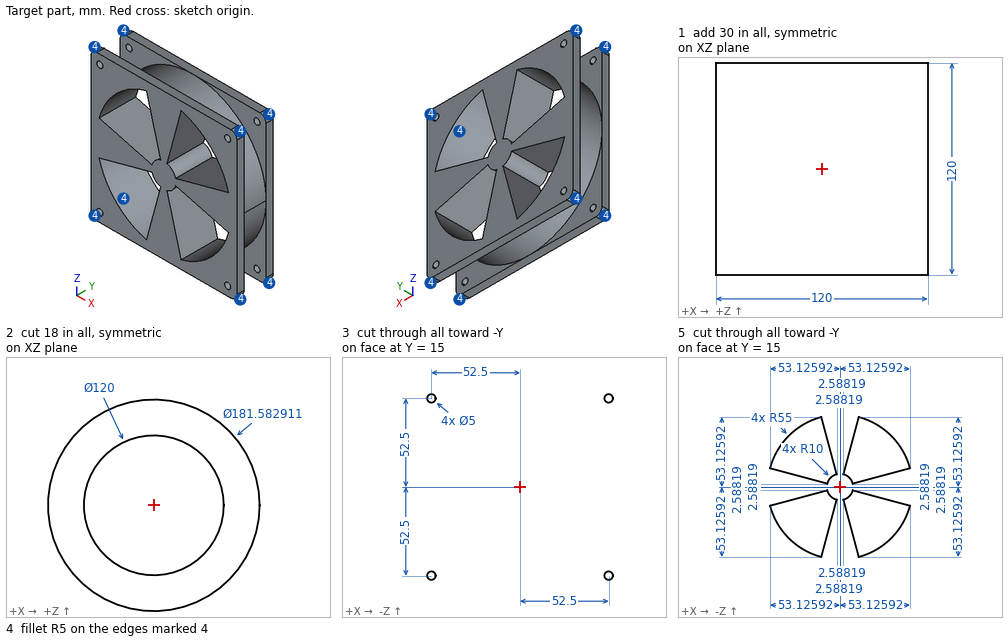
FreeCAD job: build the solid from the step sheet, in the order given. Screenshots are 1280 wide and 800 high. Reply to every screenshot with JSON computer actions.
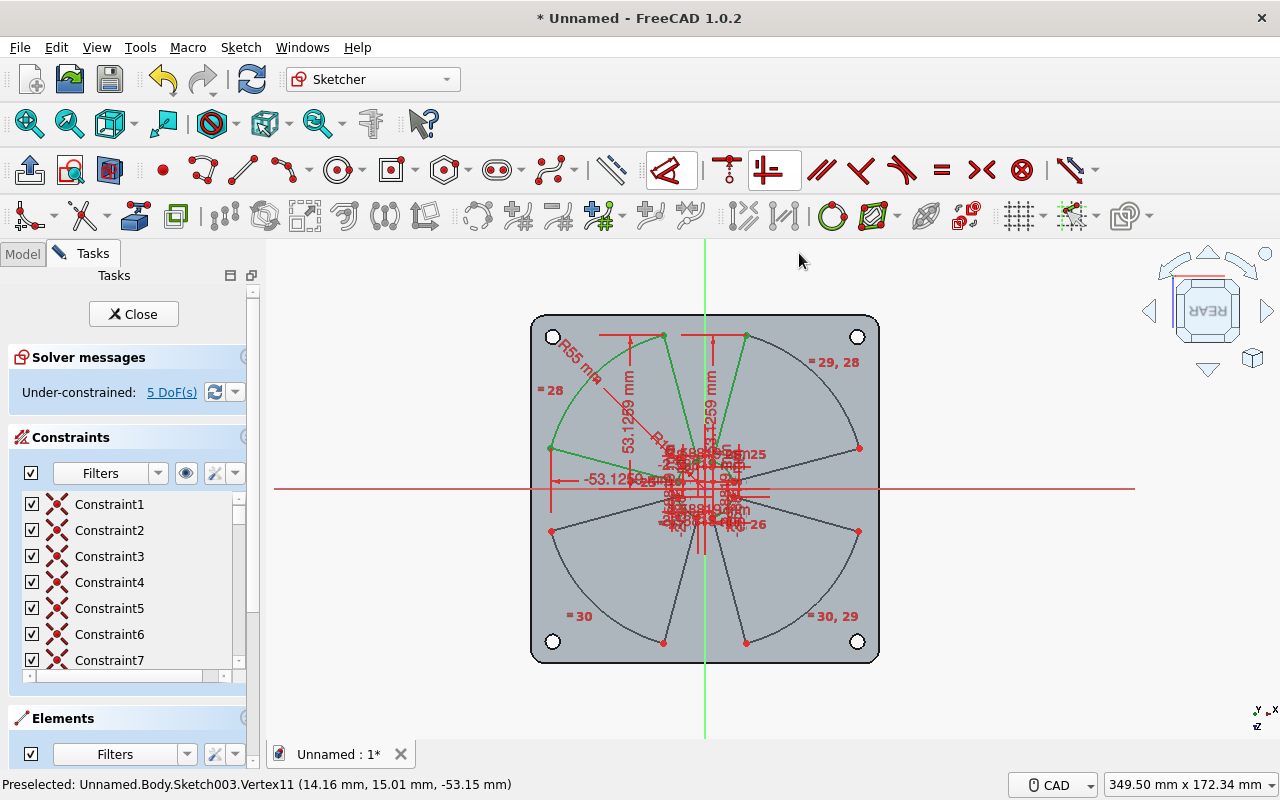
{"action": "left_click", "coordinate": [859, 449]}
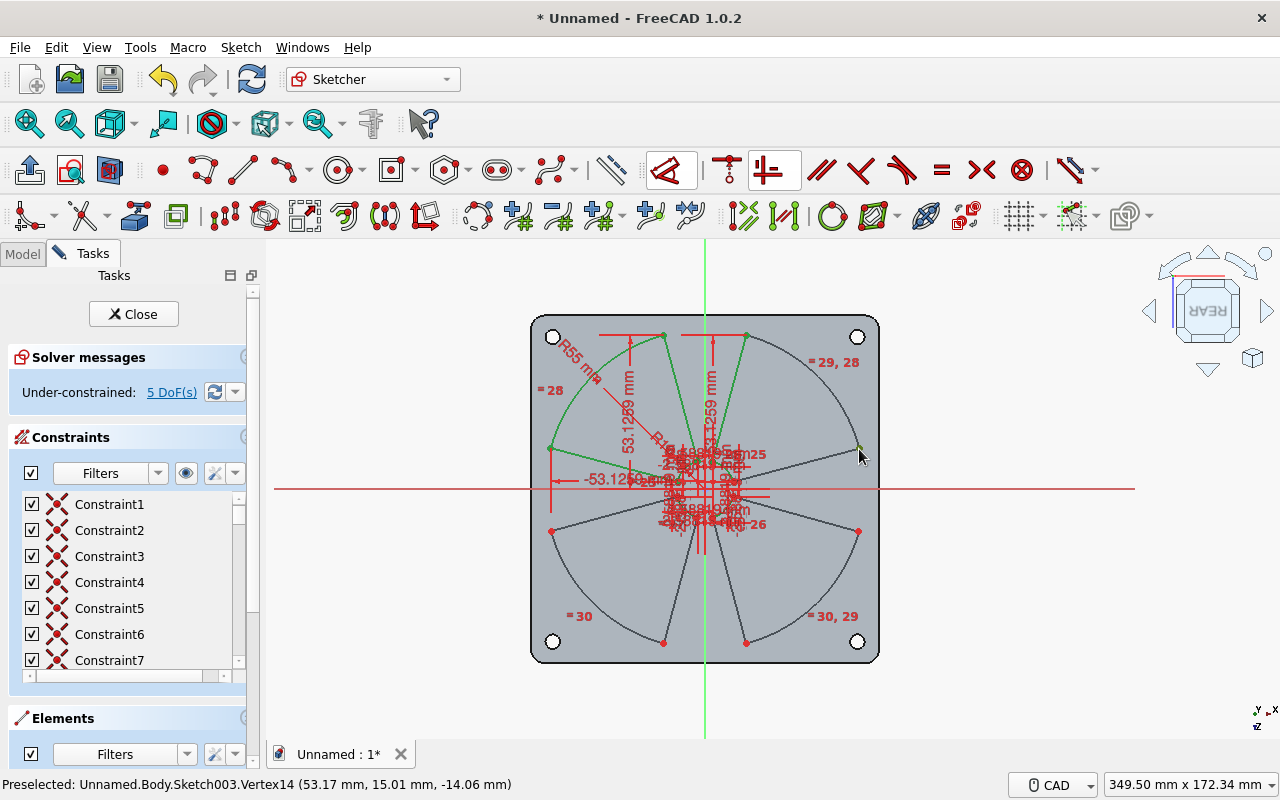
{"action": "left_click", "coordinate": [692, 170]}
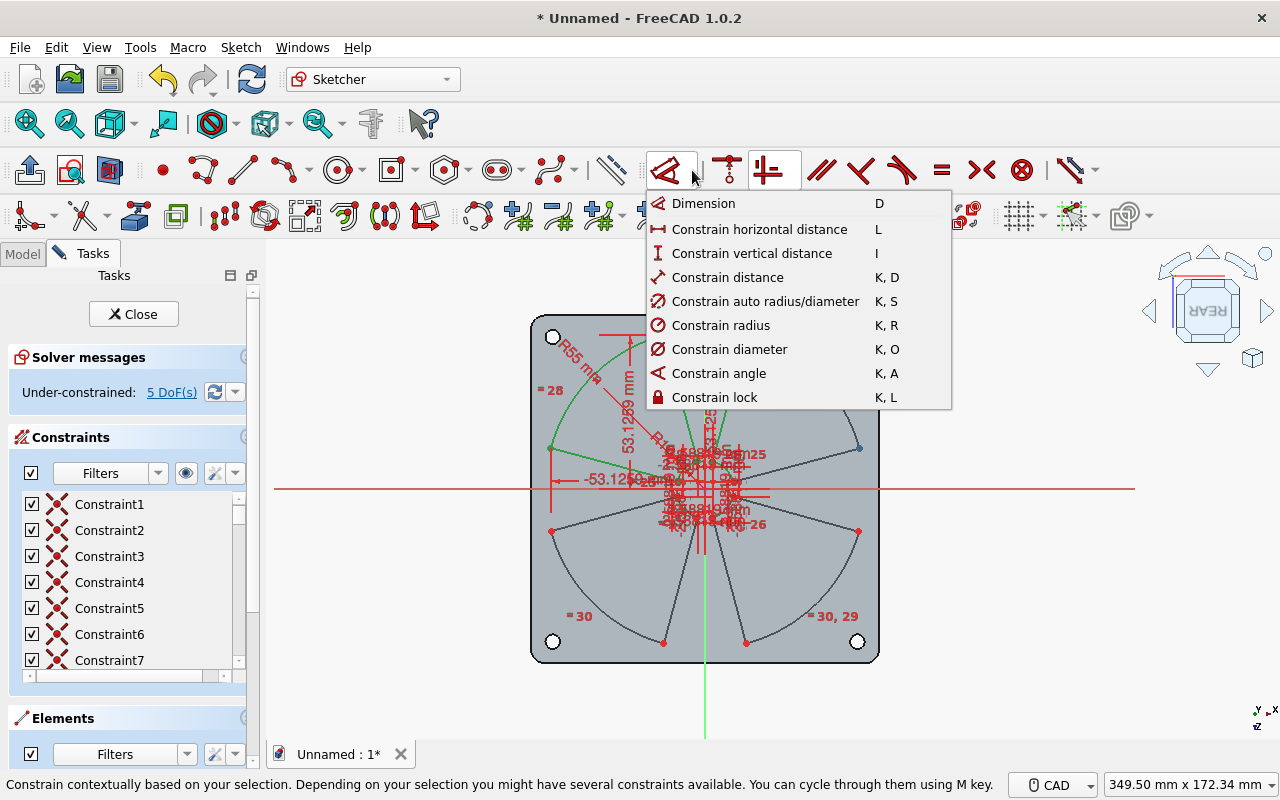
{"action": "left_click", "coordinate": [799, 229]}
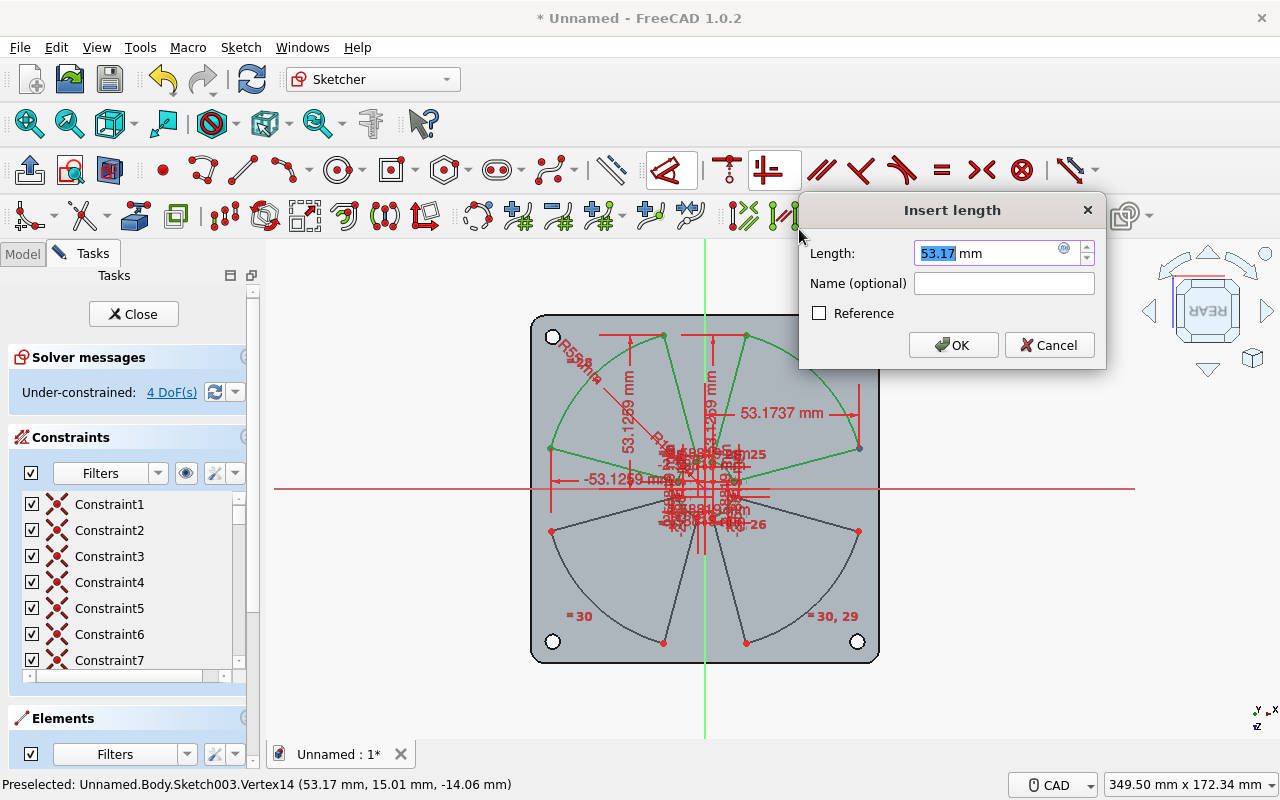
{"action": "type", "text": "53.12592"}
{"action": "key", "text": "Return"}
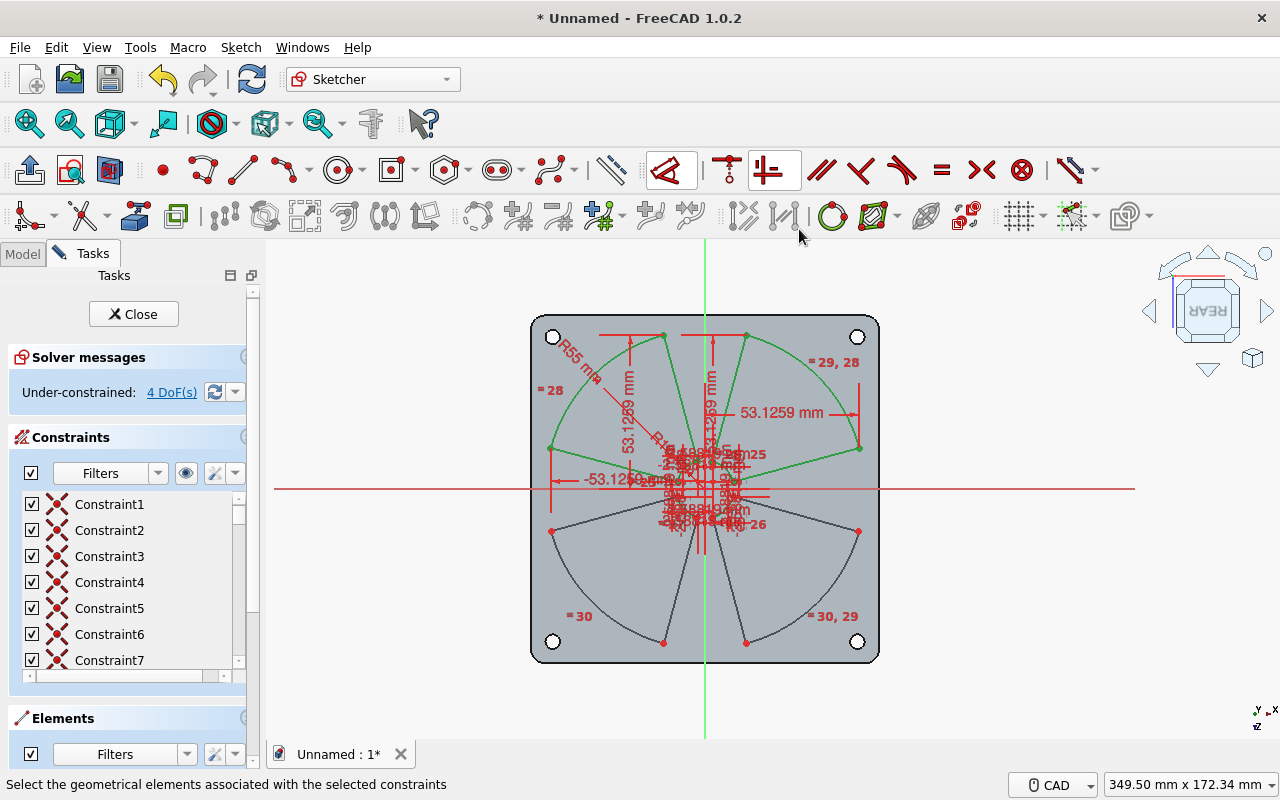
{"action": "left_click", "coordinate": [746, 644]}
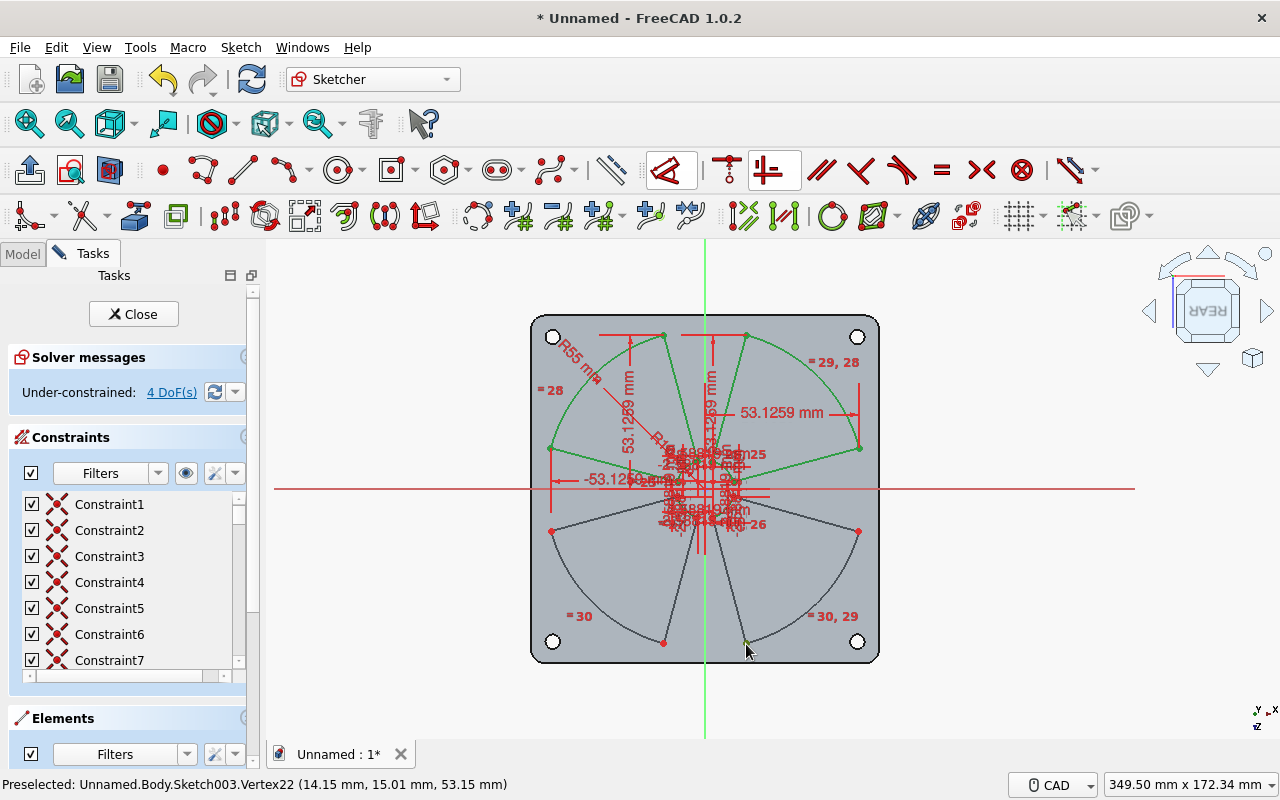
{"action": "key", "text": "i"}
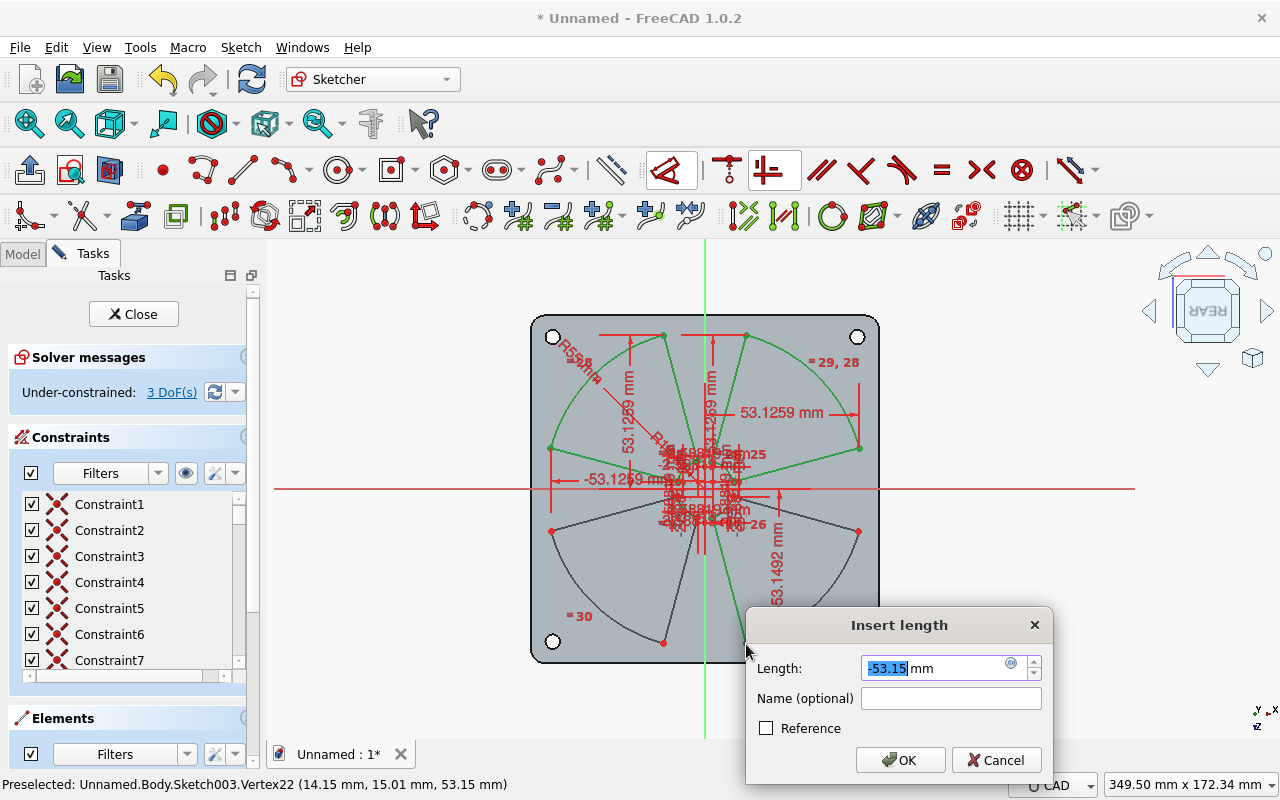
{"action": "type", "text": "-53.12592"}
{"action": "key", "text": "Return"}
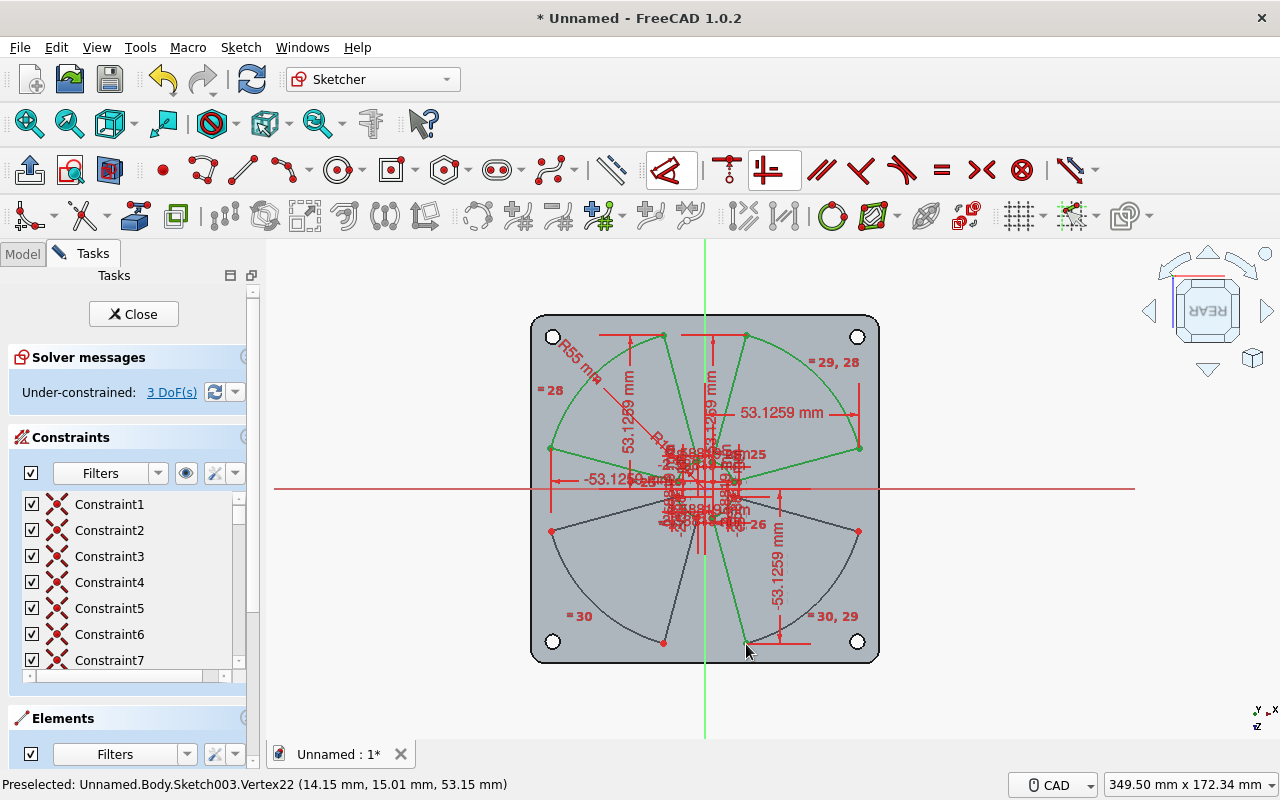
{"action": "left_click", "coordinate": [859, 532]}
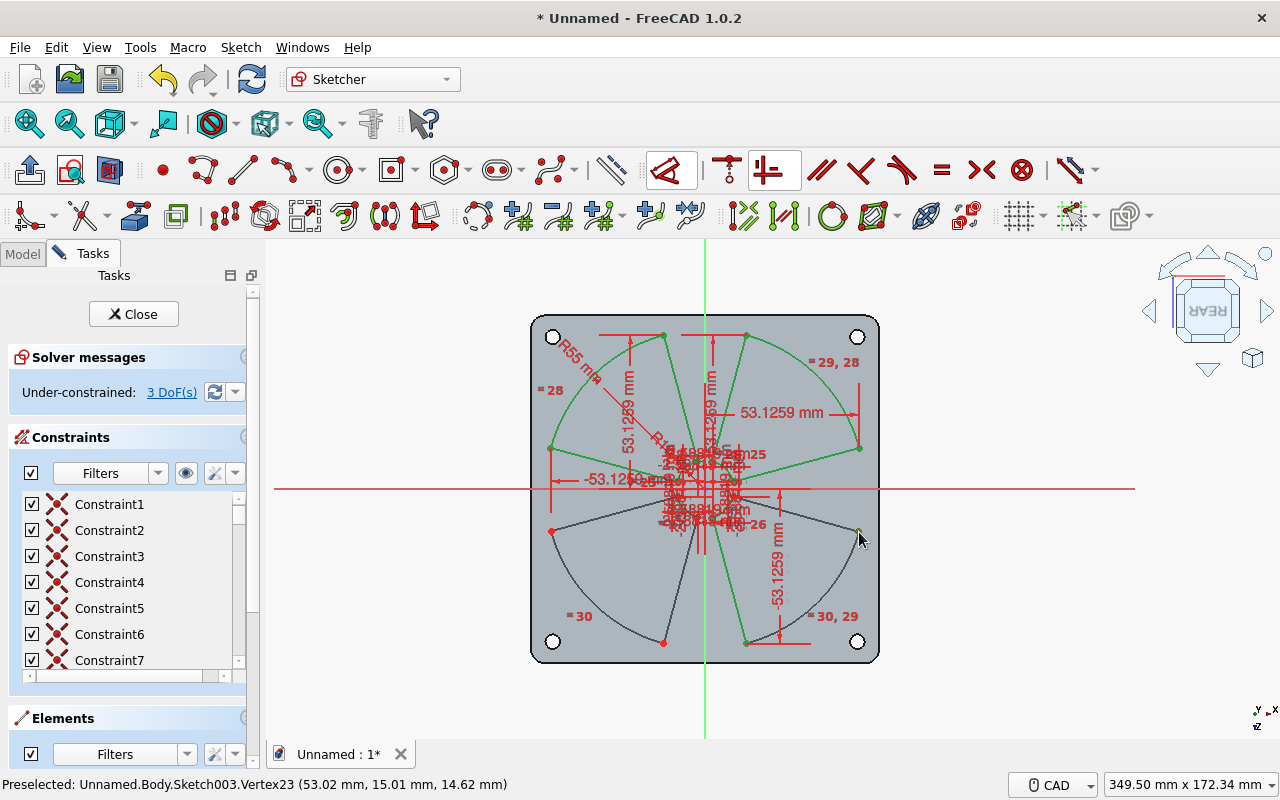
{"action": "key", "text": "l"}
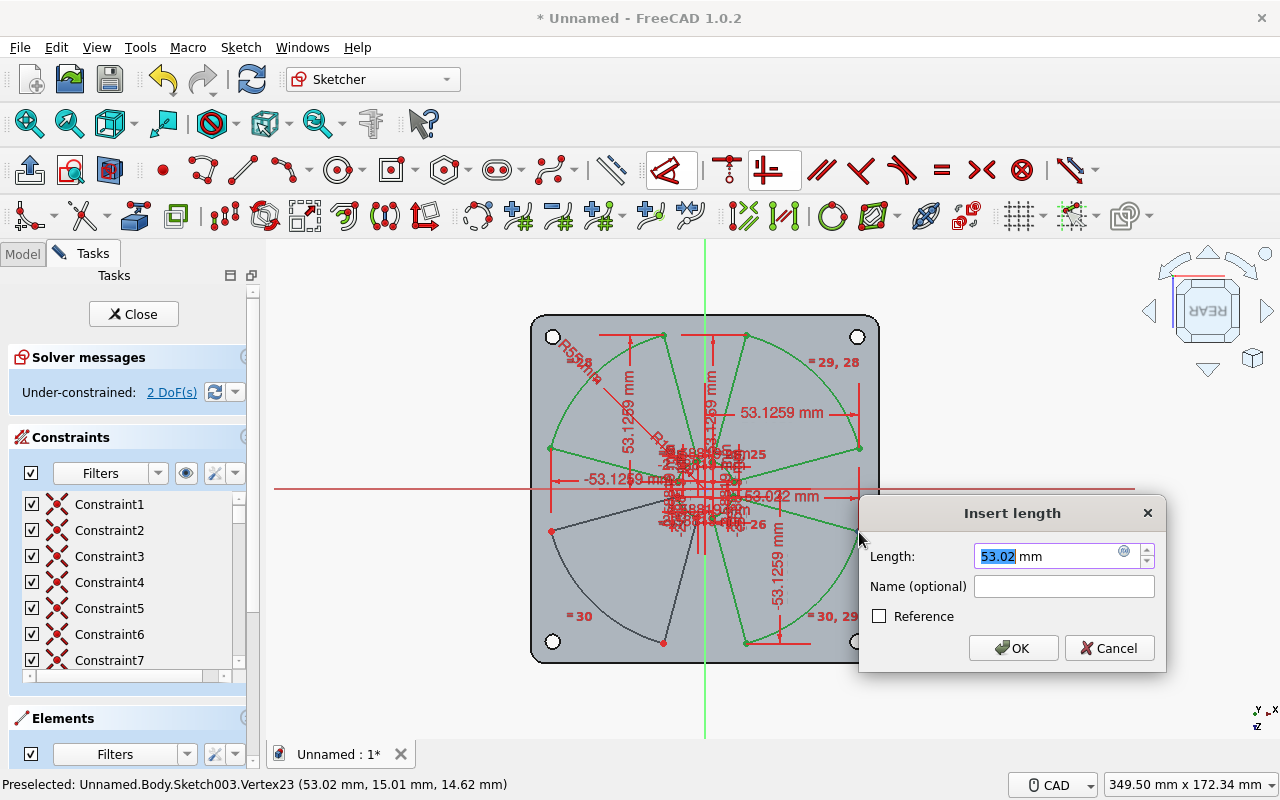
{"action": "type", "text": "53.12592"}
{"action": "key", "text": "Return"}